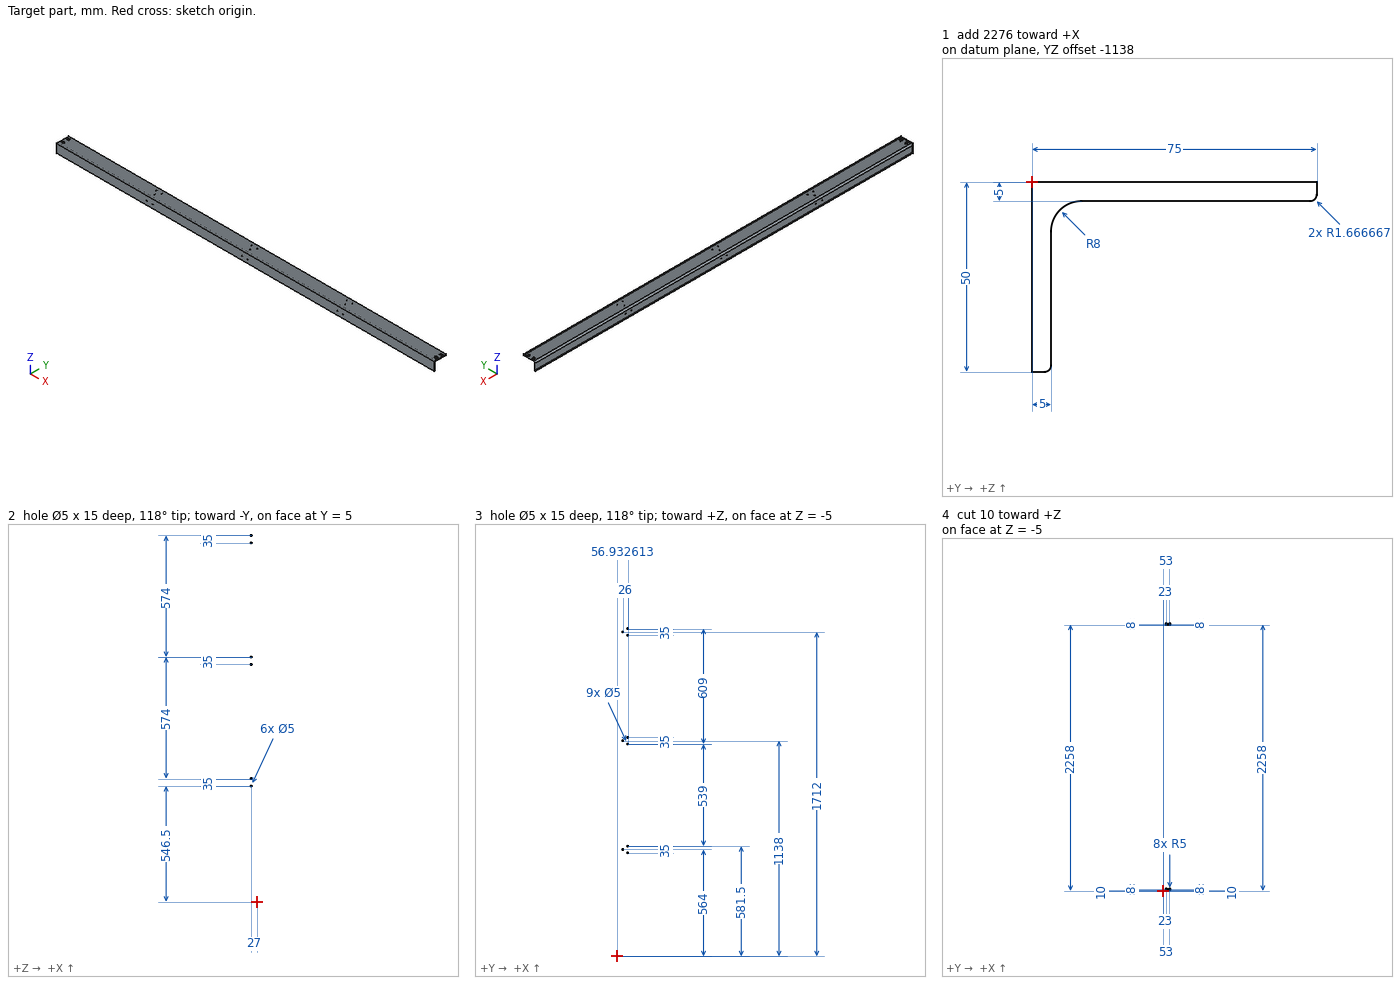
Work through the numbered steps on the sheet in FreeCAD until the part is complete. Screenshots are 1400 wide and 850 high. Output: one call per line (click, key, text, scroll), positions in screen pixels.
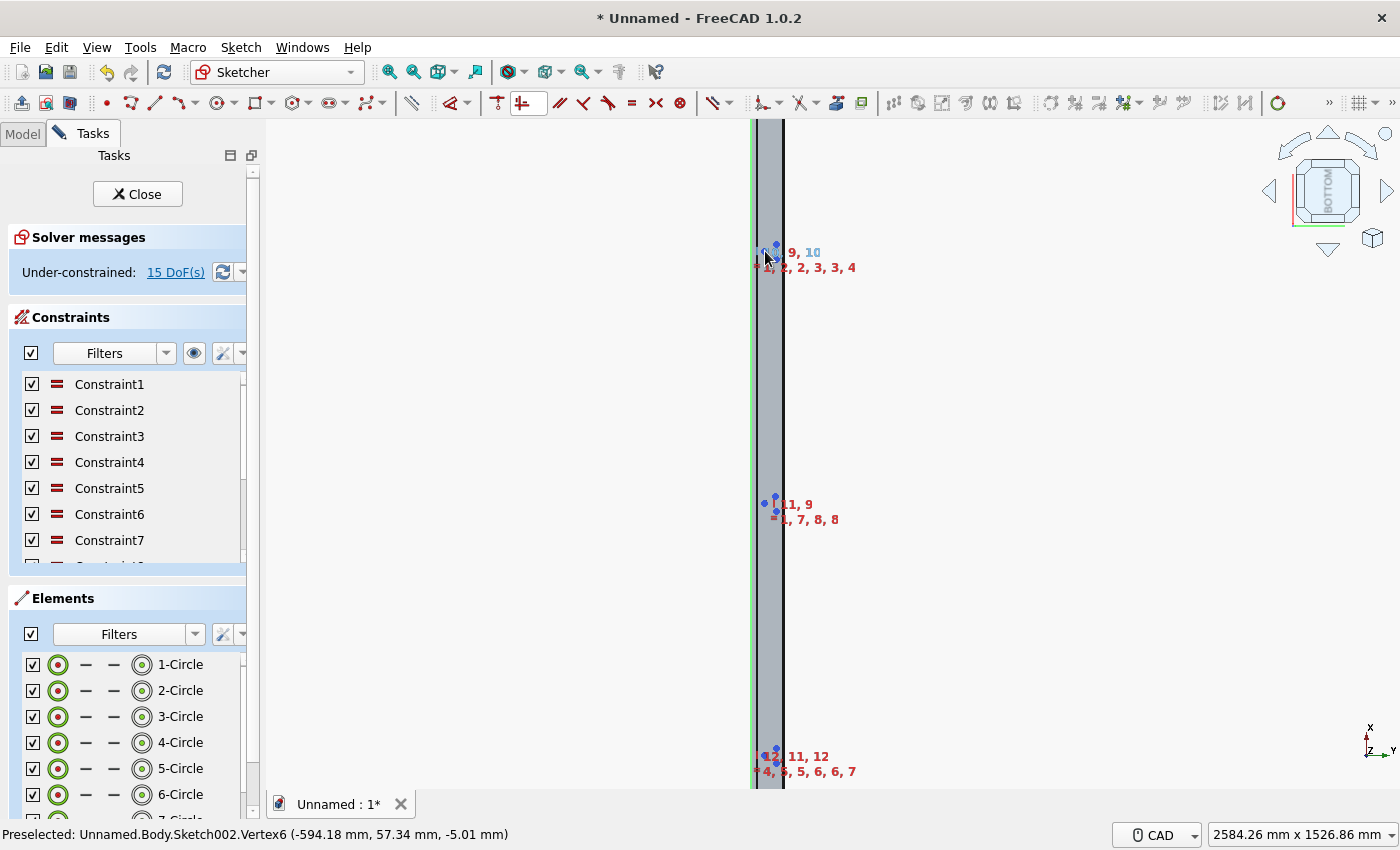
scroll(765, 251, up, 4)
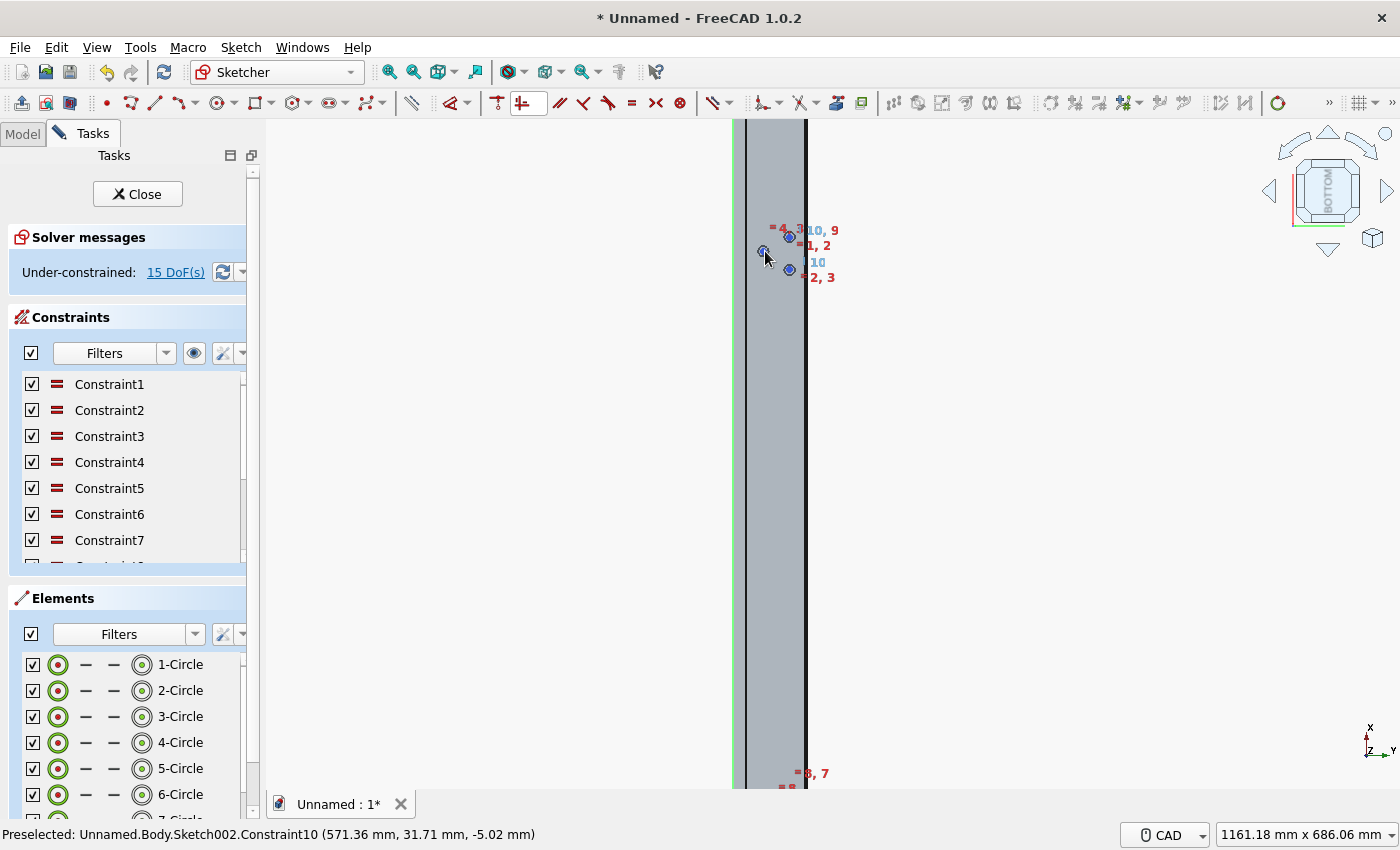
click(763, 251)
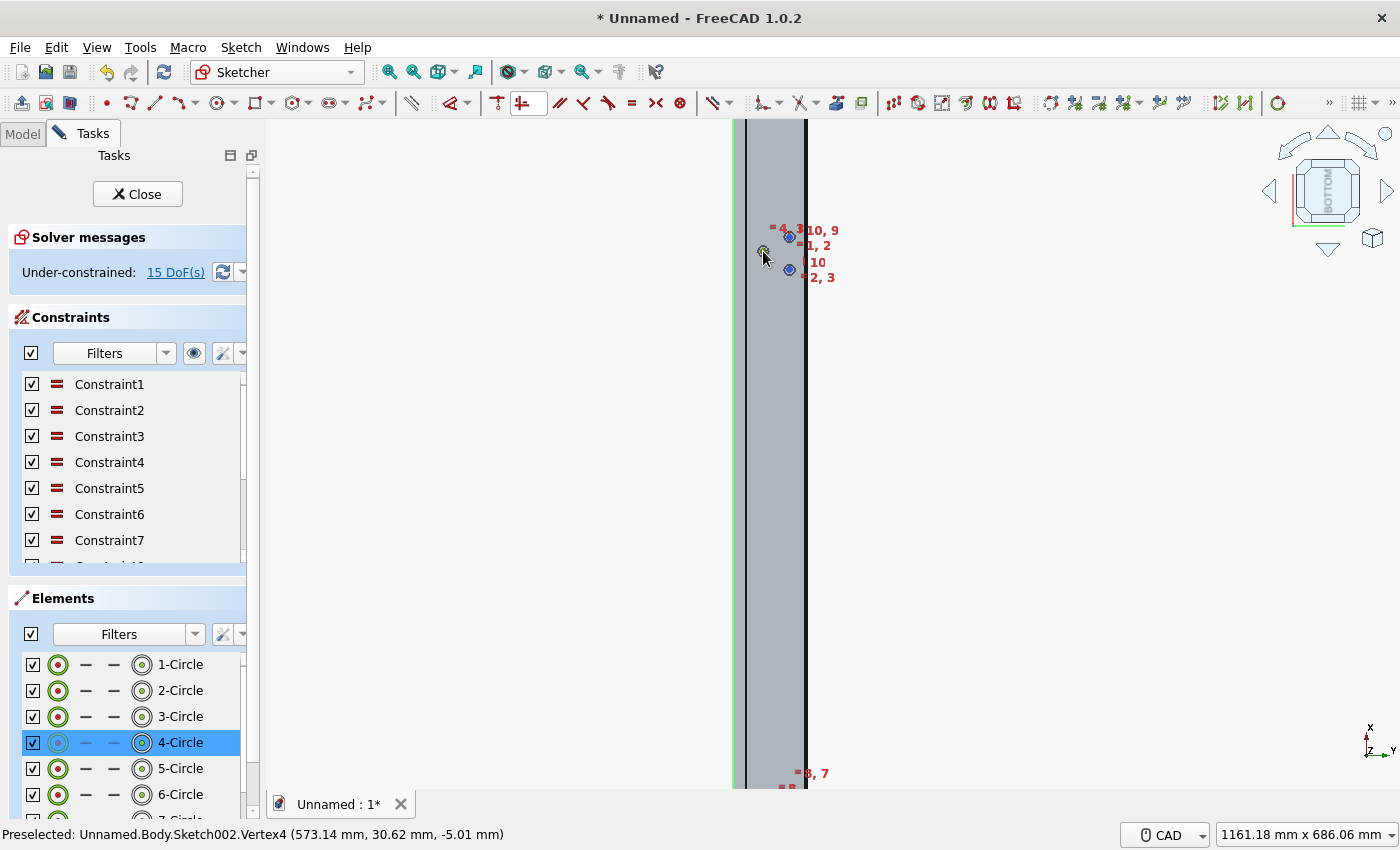
scroll(765, 250, down, 7)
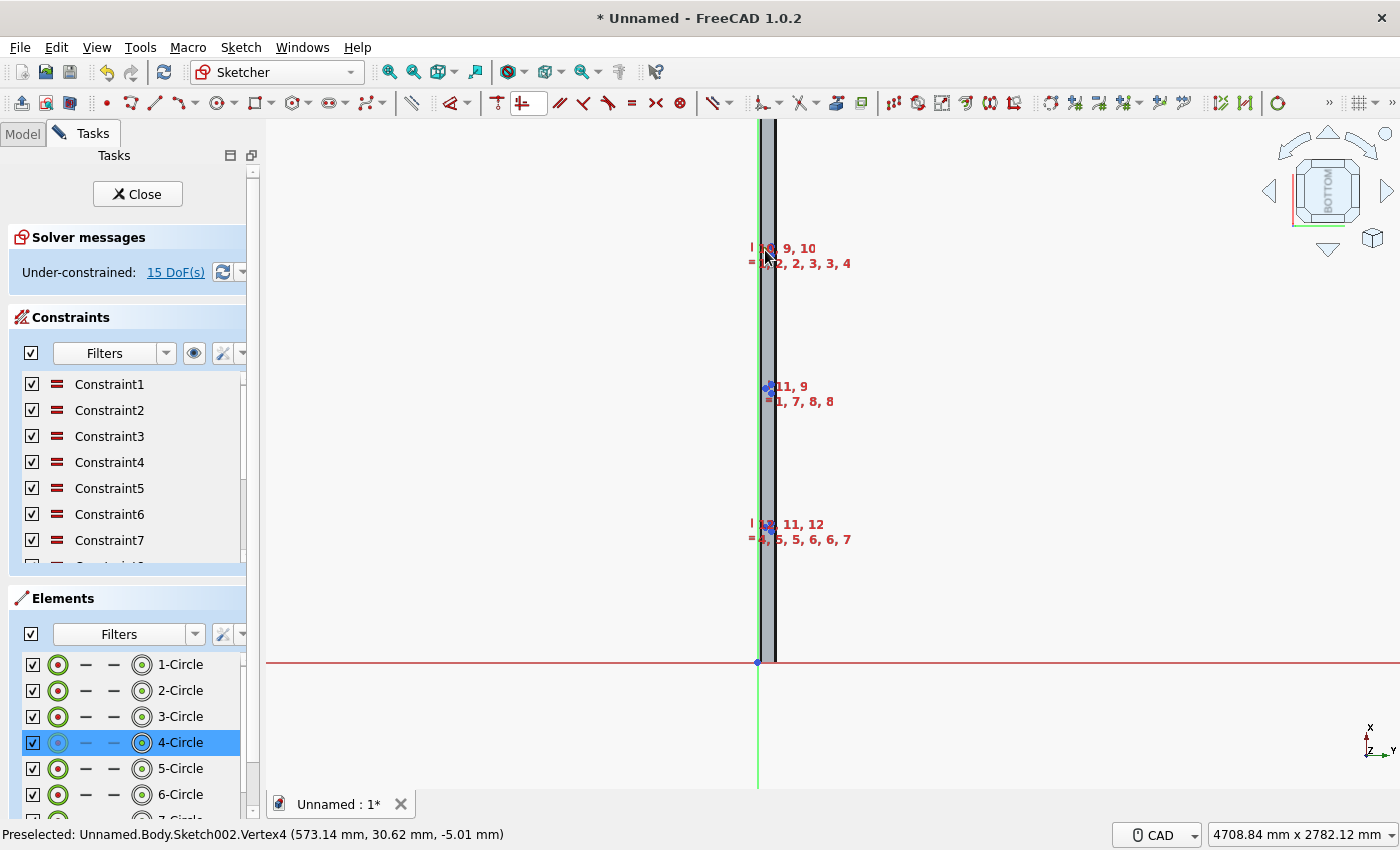
scroll(765, 527, up, 3)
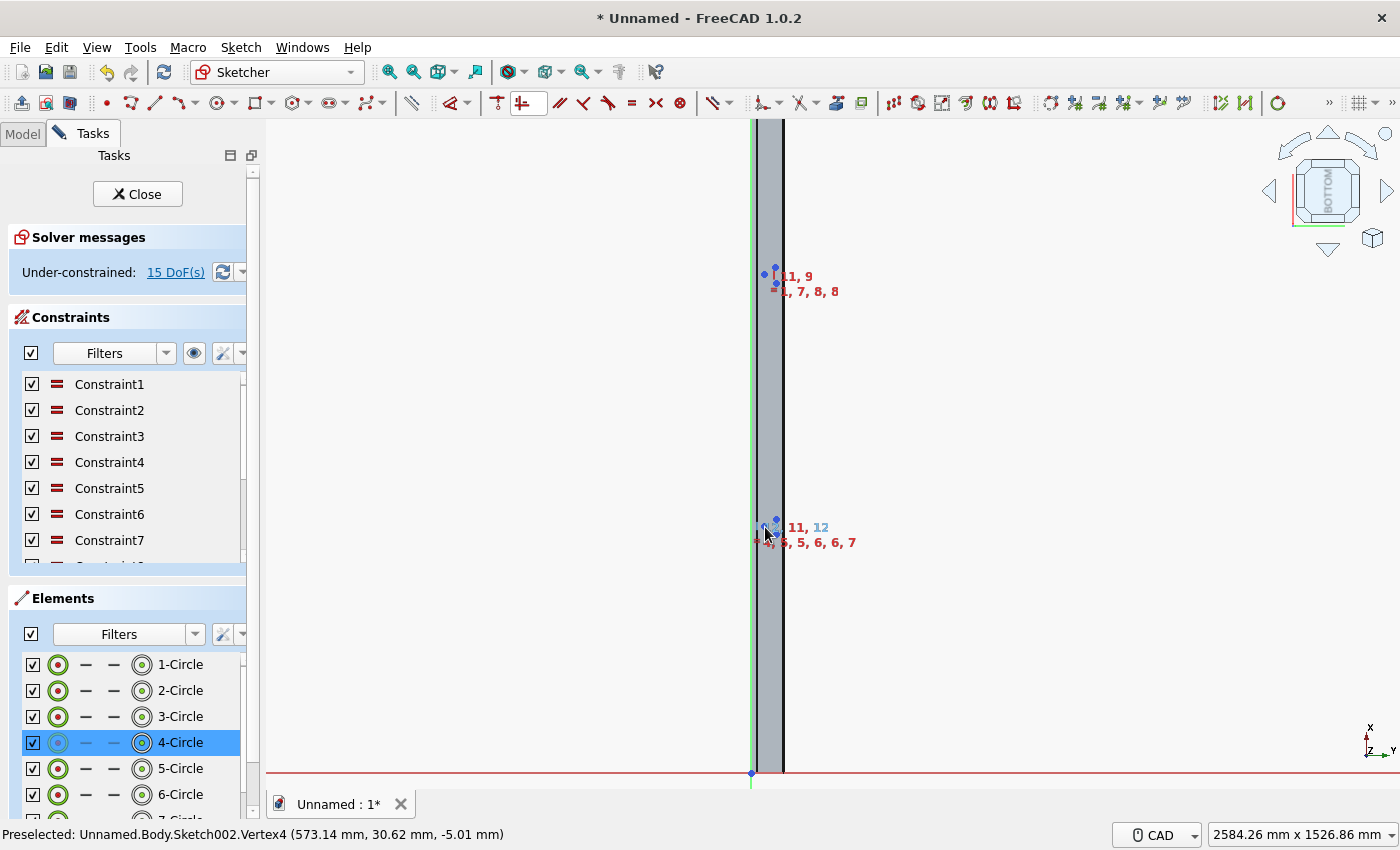
scroll(765, 527, up, 4)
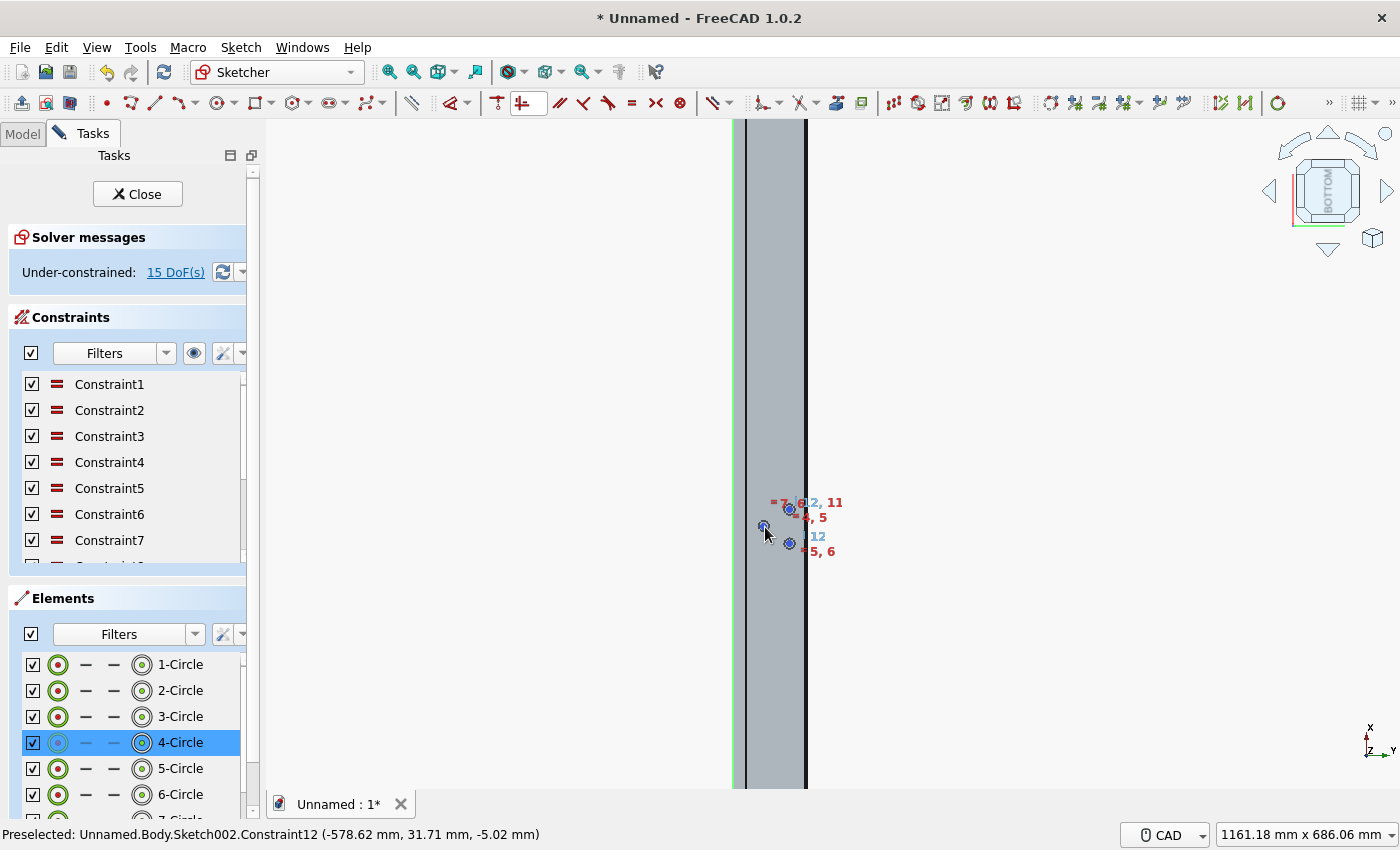
click(764, 526)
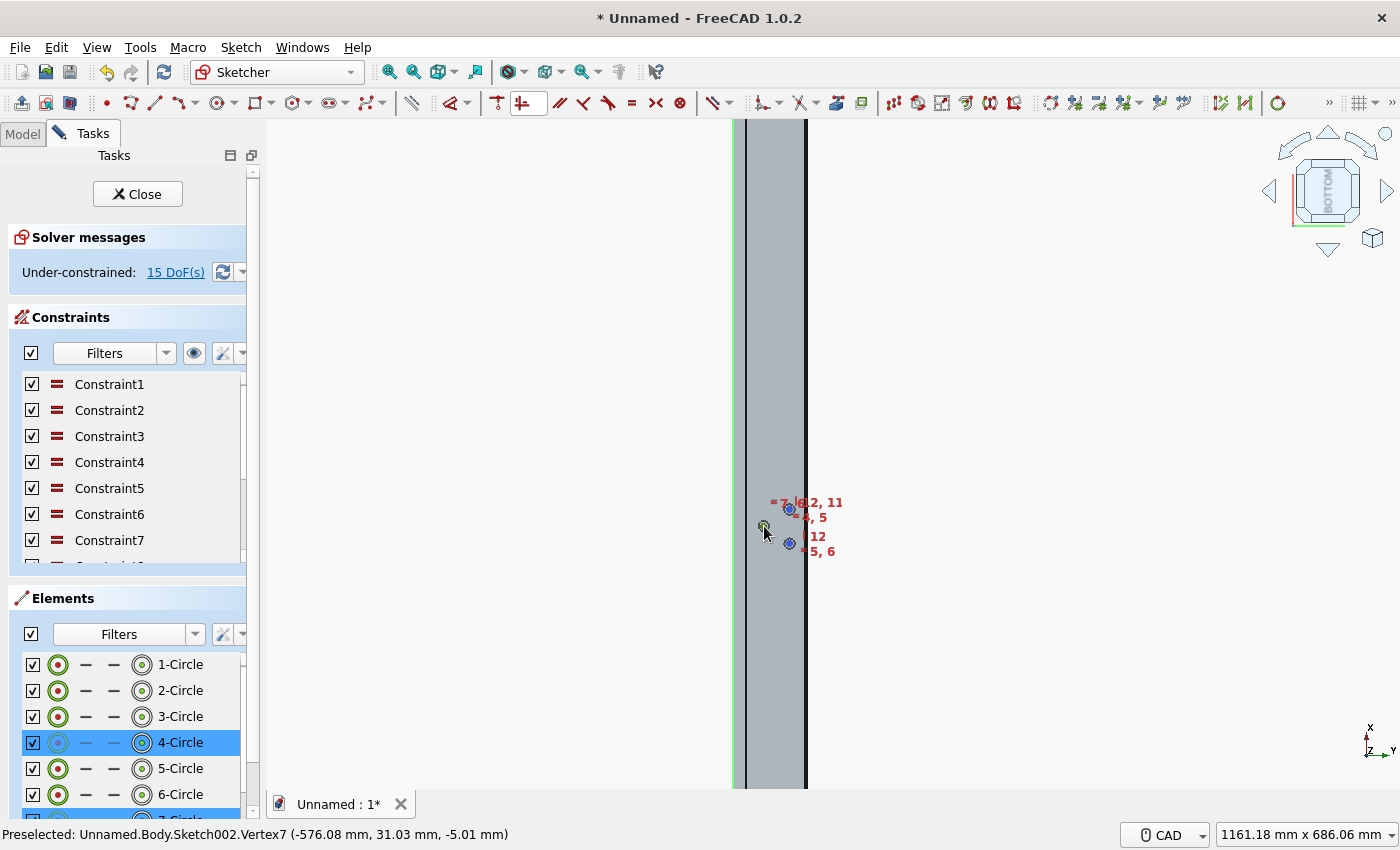
click(542, 104)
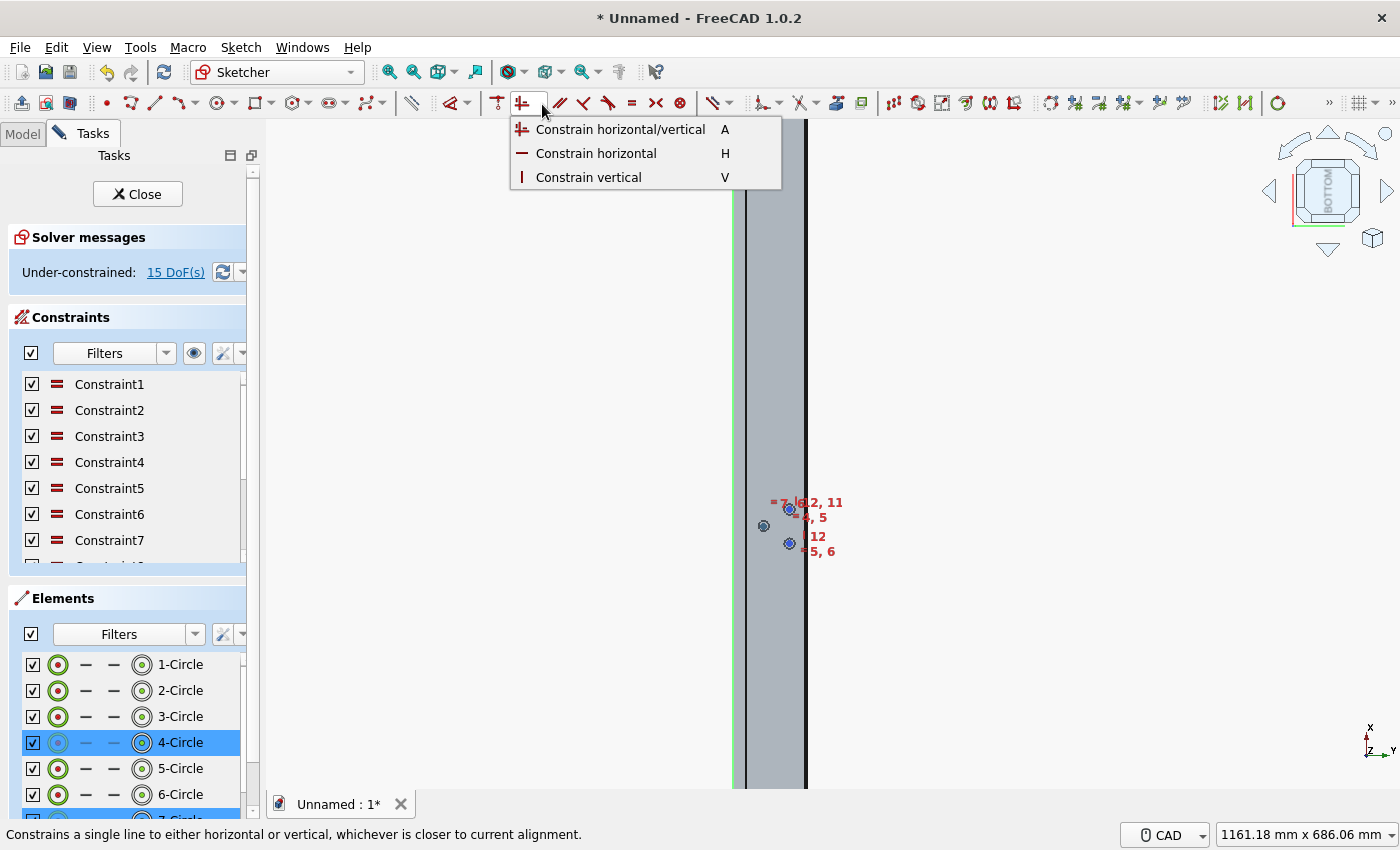
click(646, 177)